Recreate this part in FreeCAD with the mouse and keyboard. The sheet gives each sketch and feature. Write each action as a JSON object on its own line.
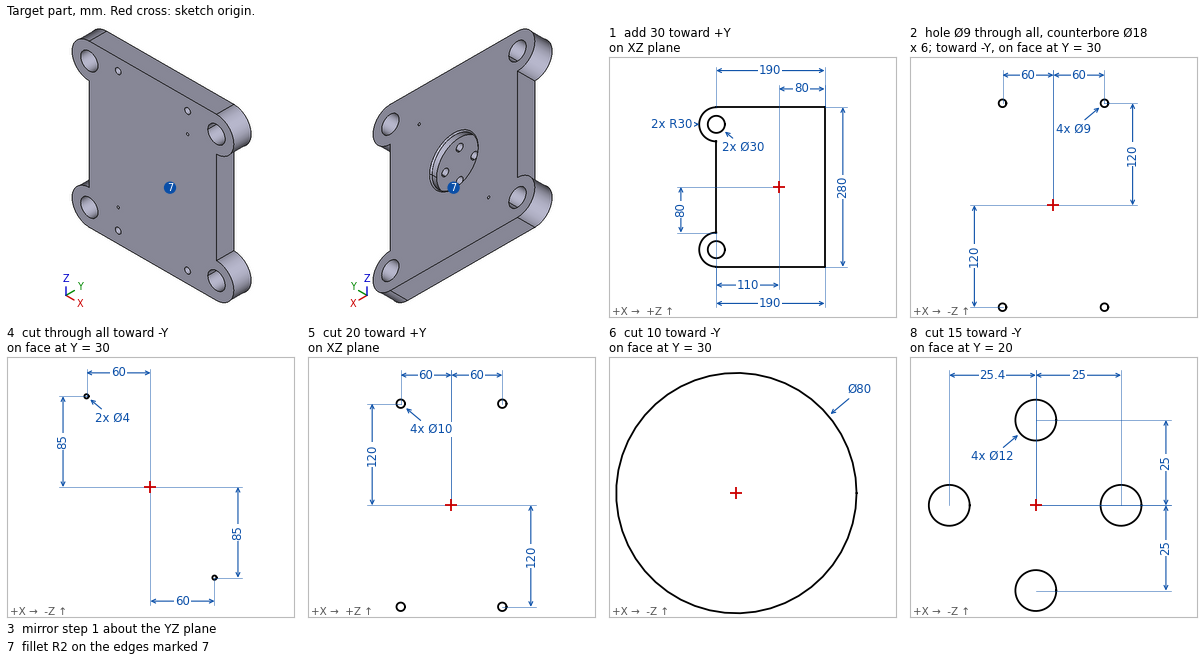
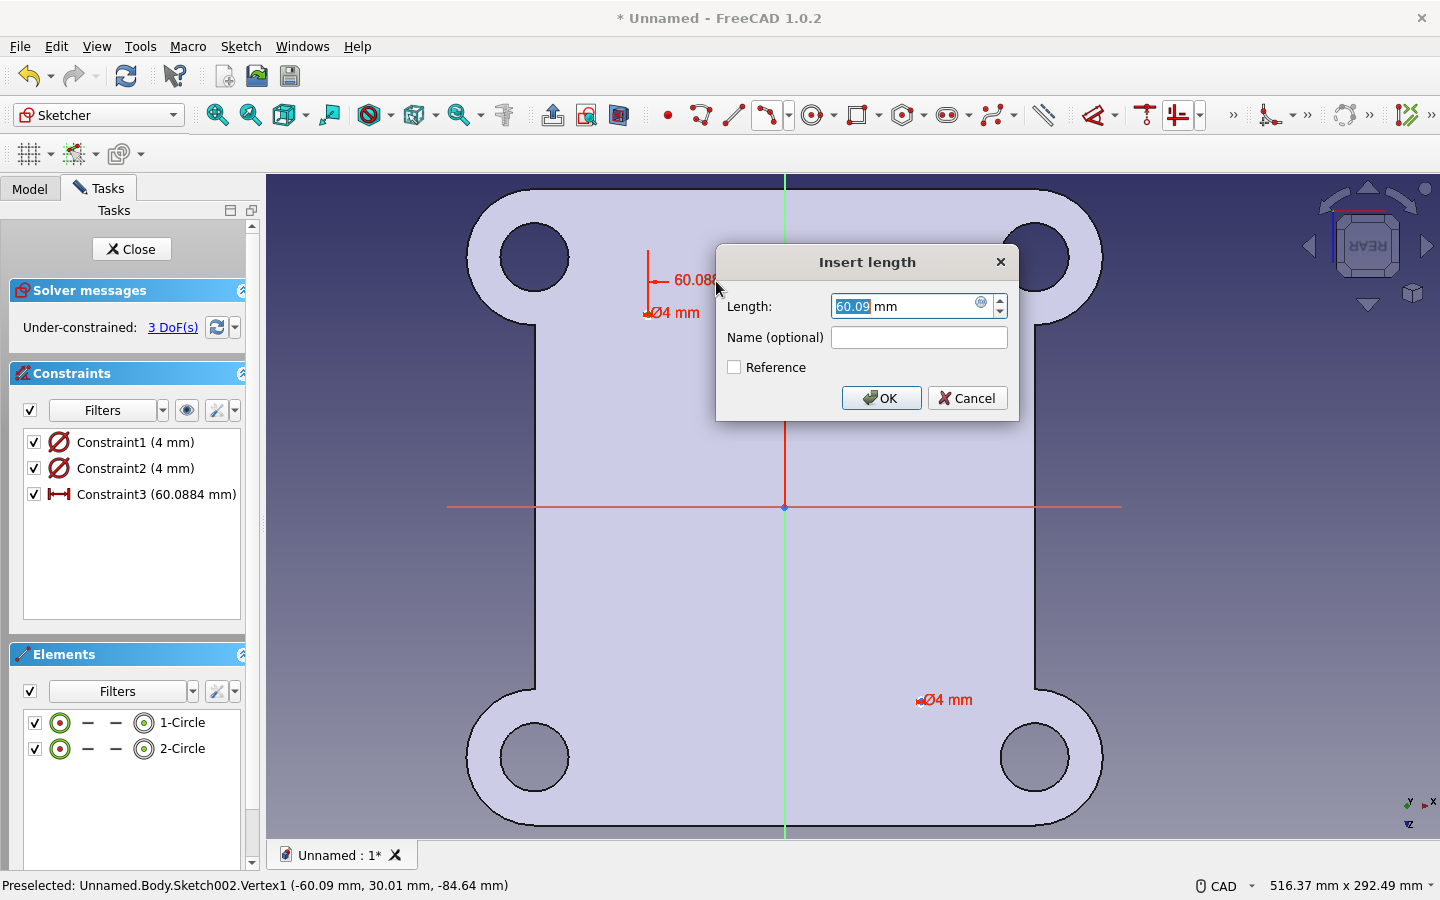
{"action": "type", "text": "60"}
{"action": "key", "text": "Return"}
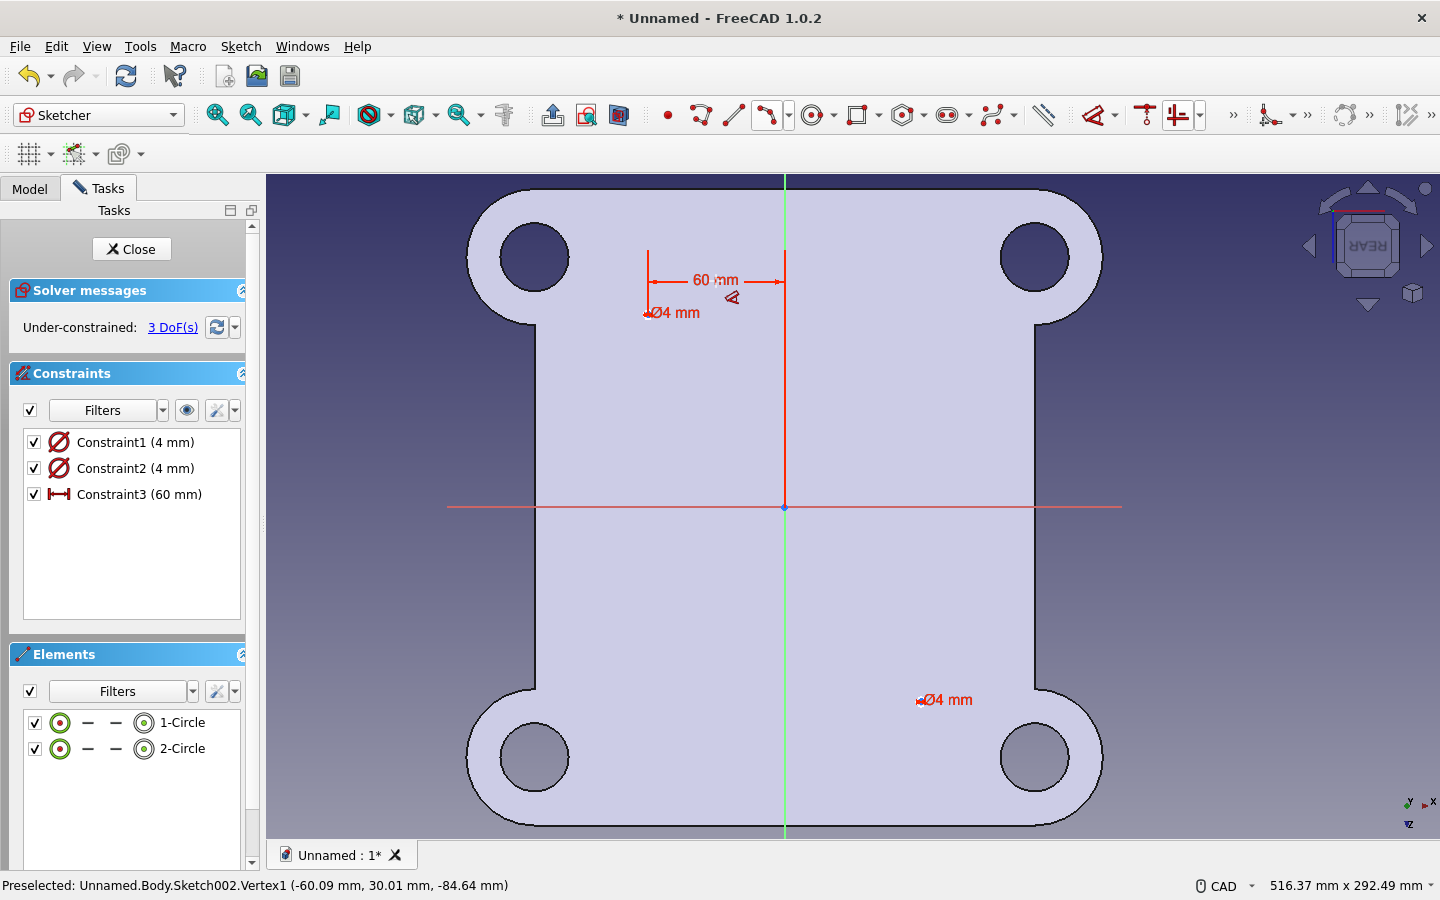
{"action": "left_click", "coordinate": [648, 315]}
{"action": "left_click", "coordinate": [614, 411]}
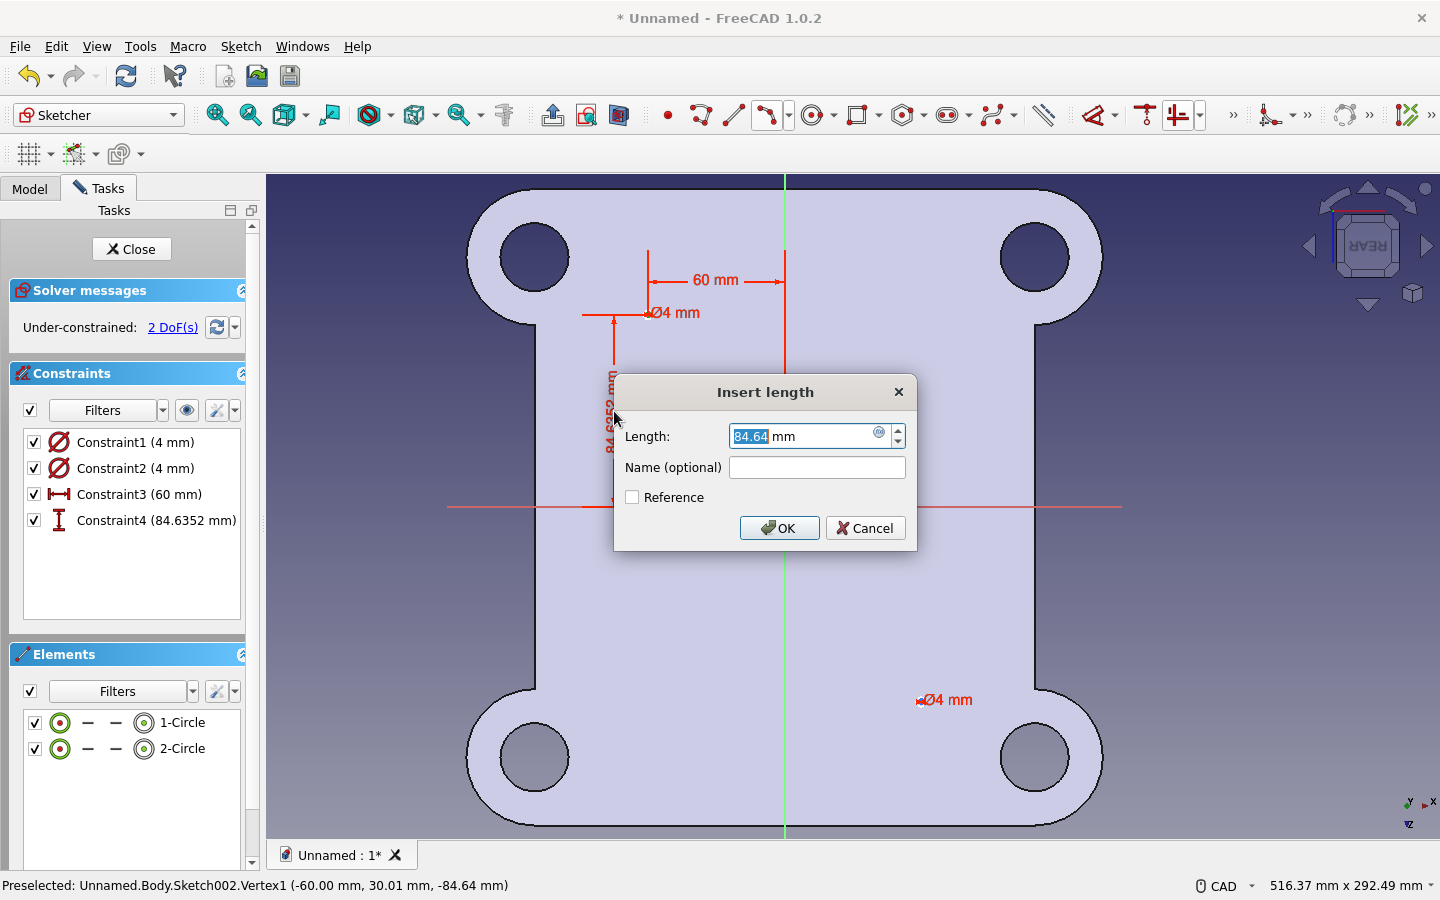
{"action": "type", "text": "85"}
{"action": "key", "text": "Return"}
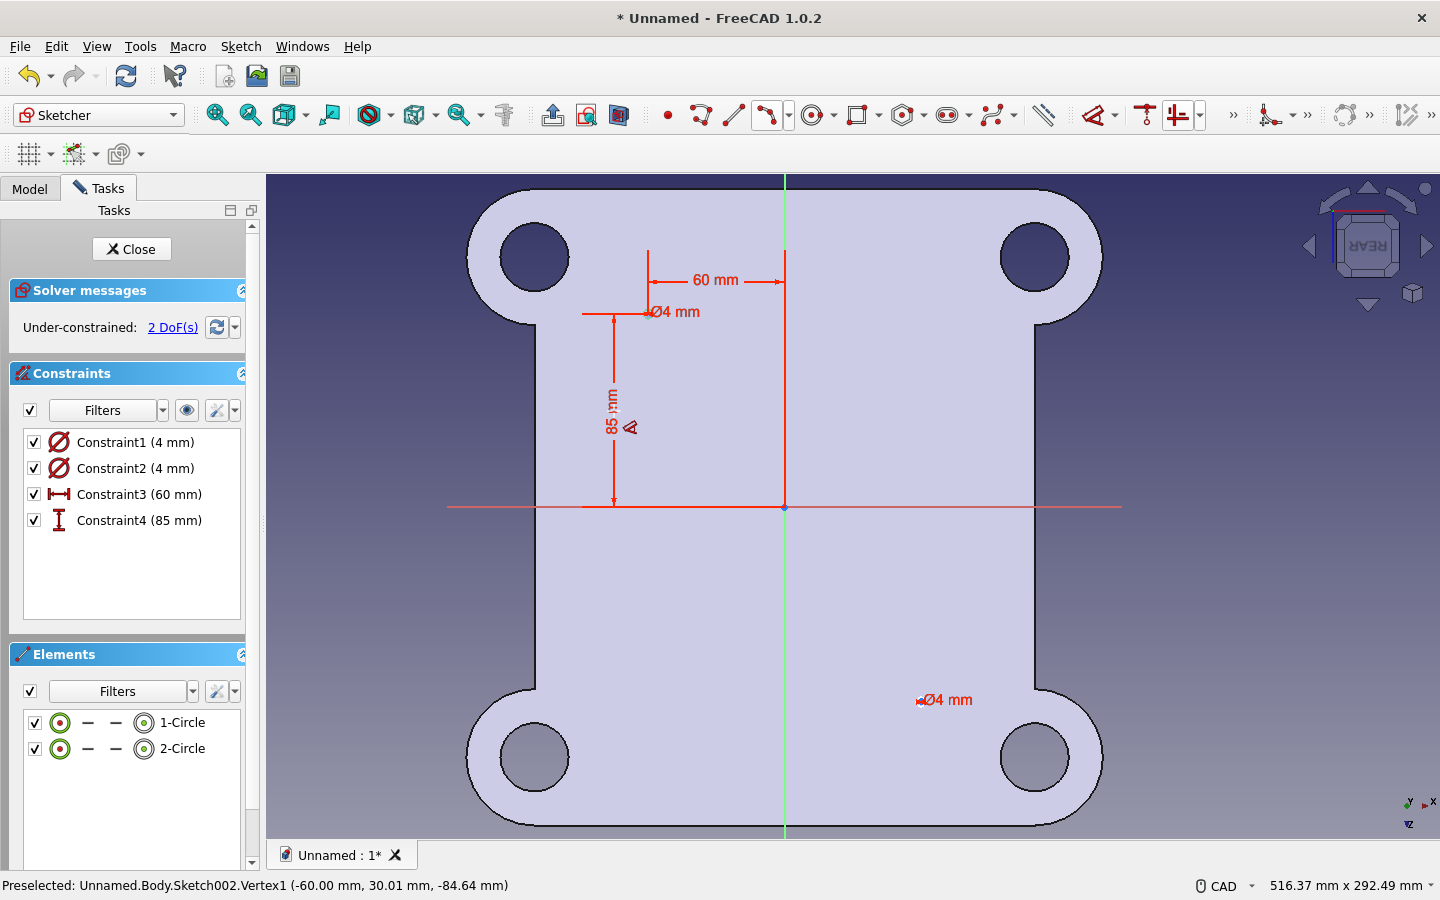
{"action": "left_click", "coordinate": [921, 702]}
{"action": "left_click", "coordinate": [853, 736]}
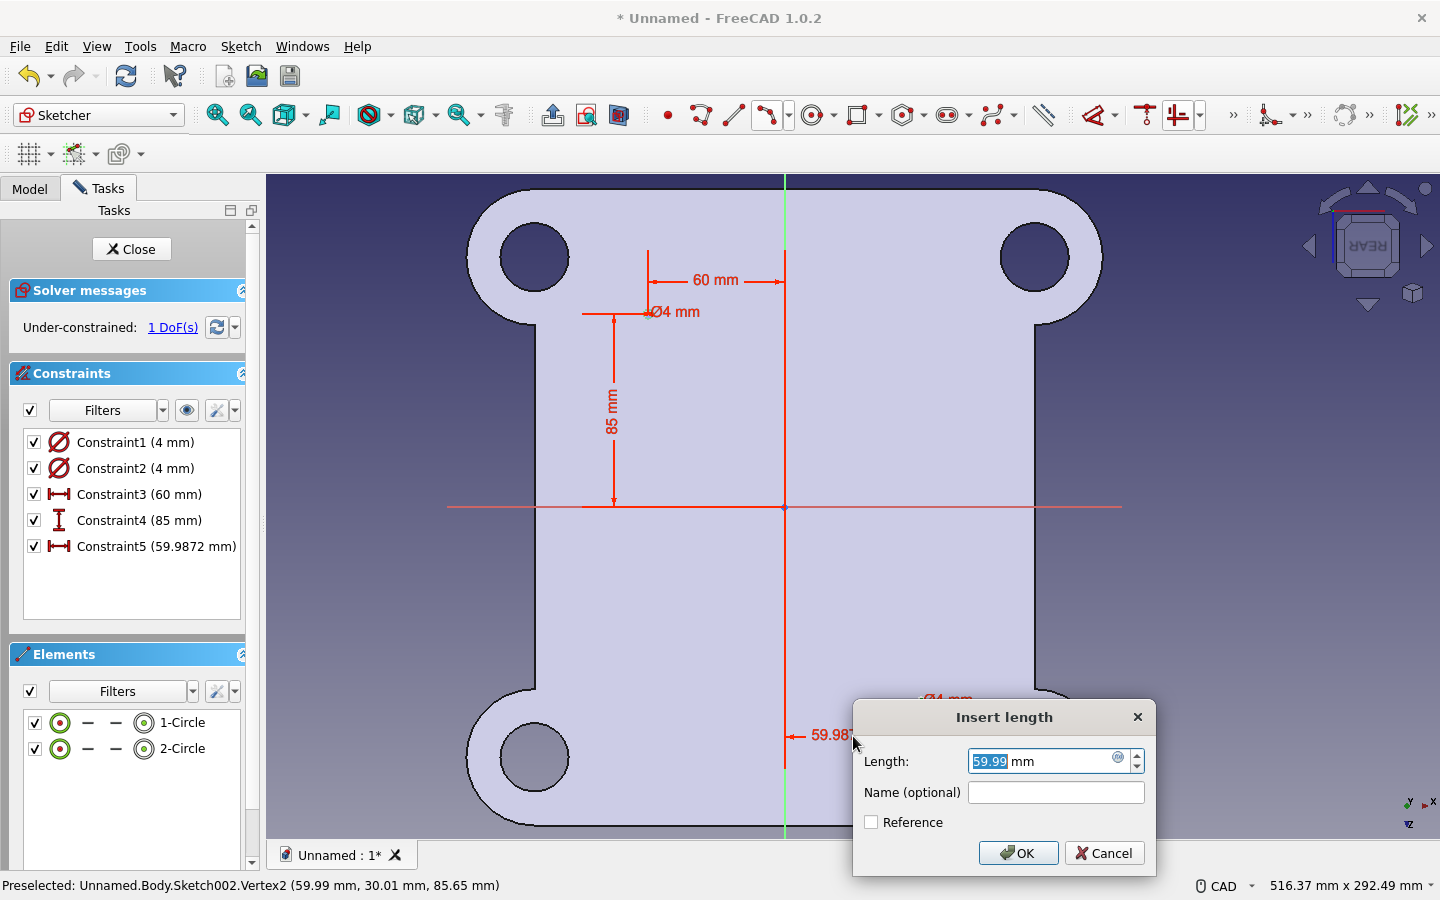
{"action": "type", "text": "60"}
{"action": "key", "text": "Return"}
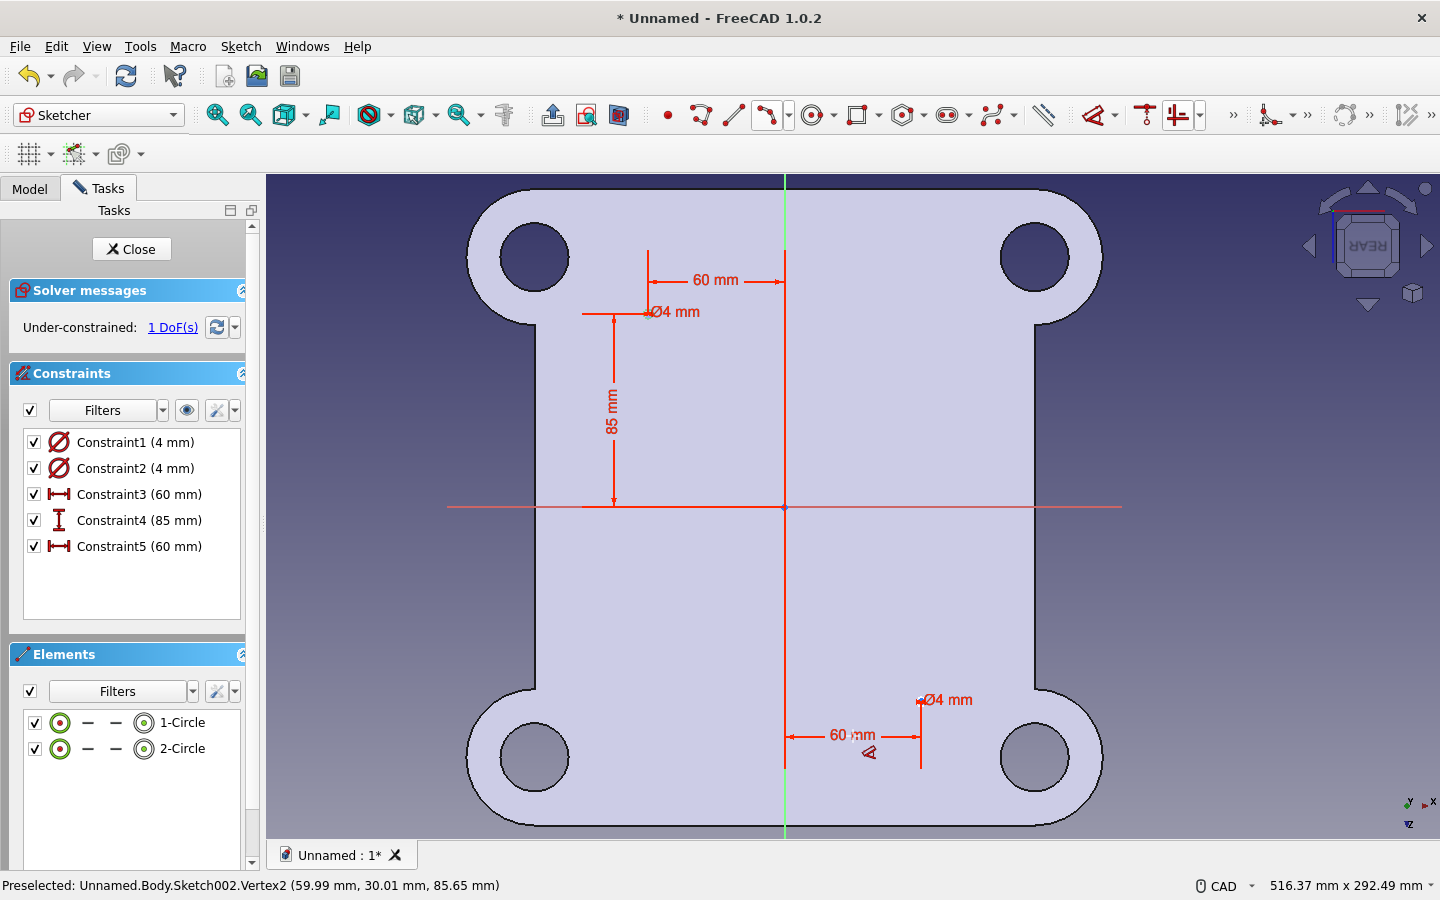
{"action": "left_click", "coordinate": [921, 702]}
{"action": "left_click", "coordinate": [955, 605]}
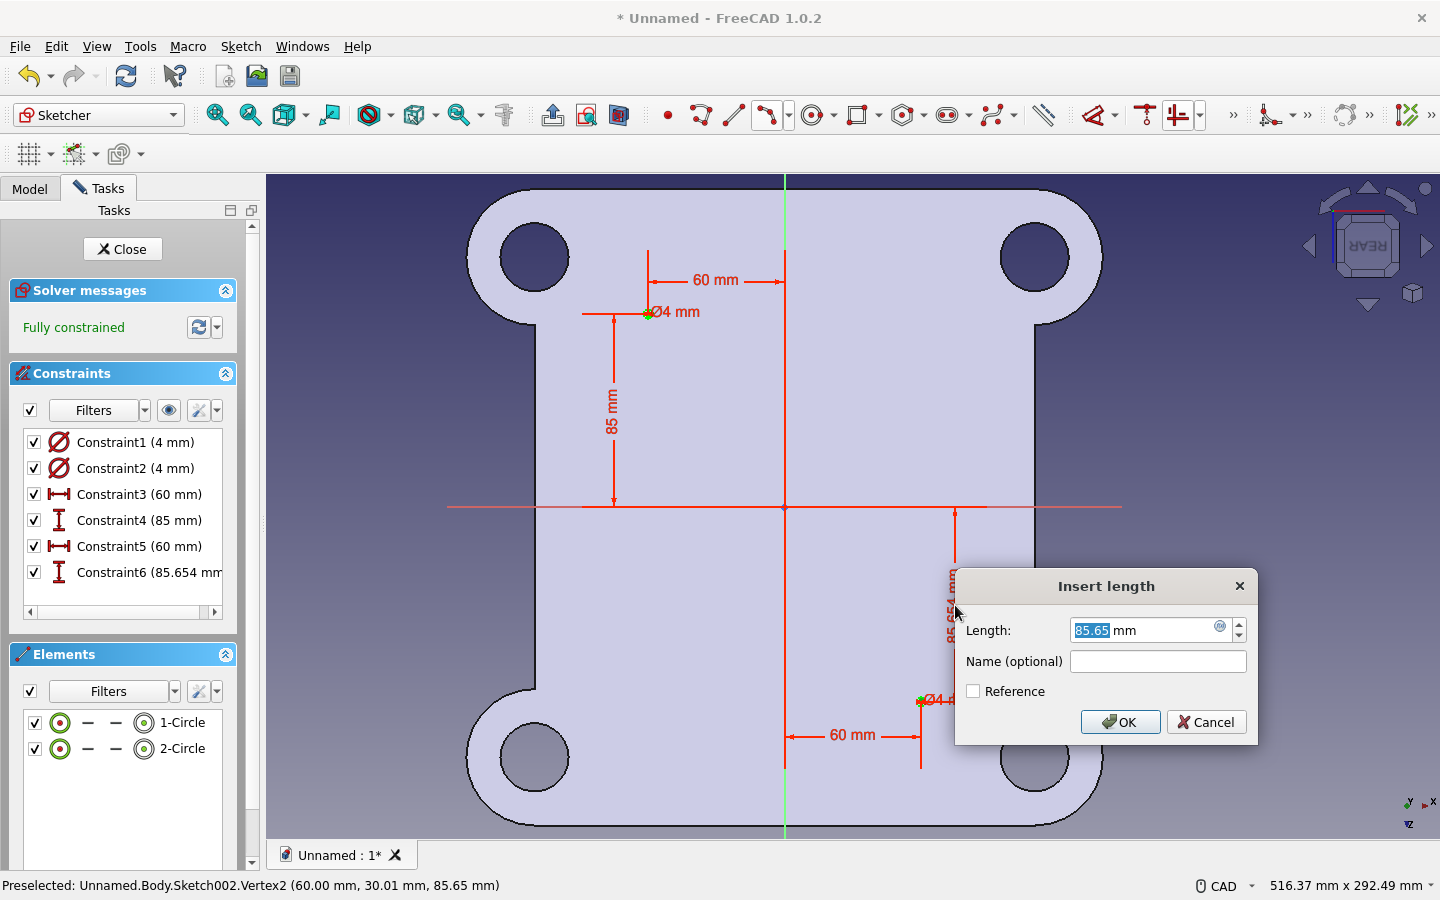
{"action": "type", "text": "85"}
{"action": "key", "text": "Return"}
{"action": "key", "text": "Escape"}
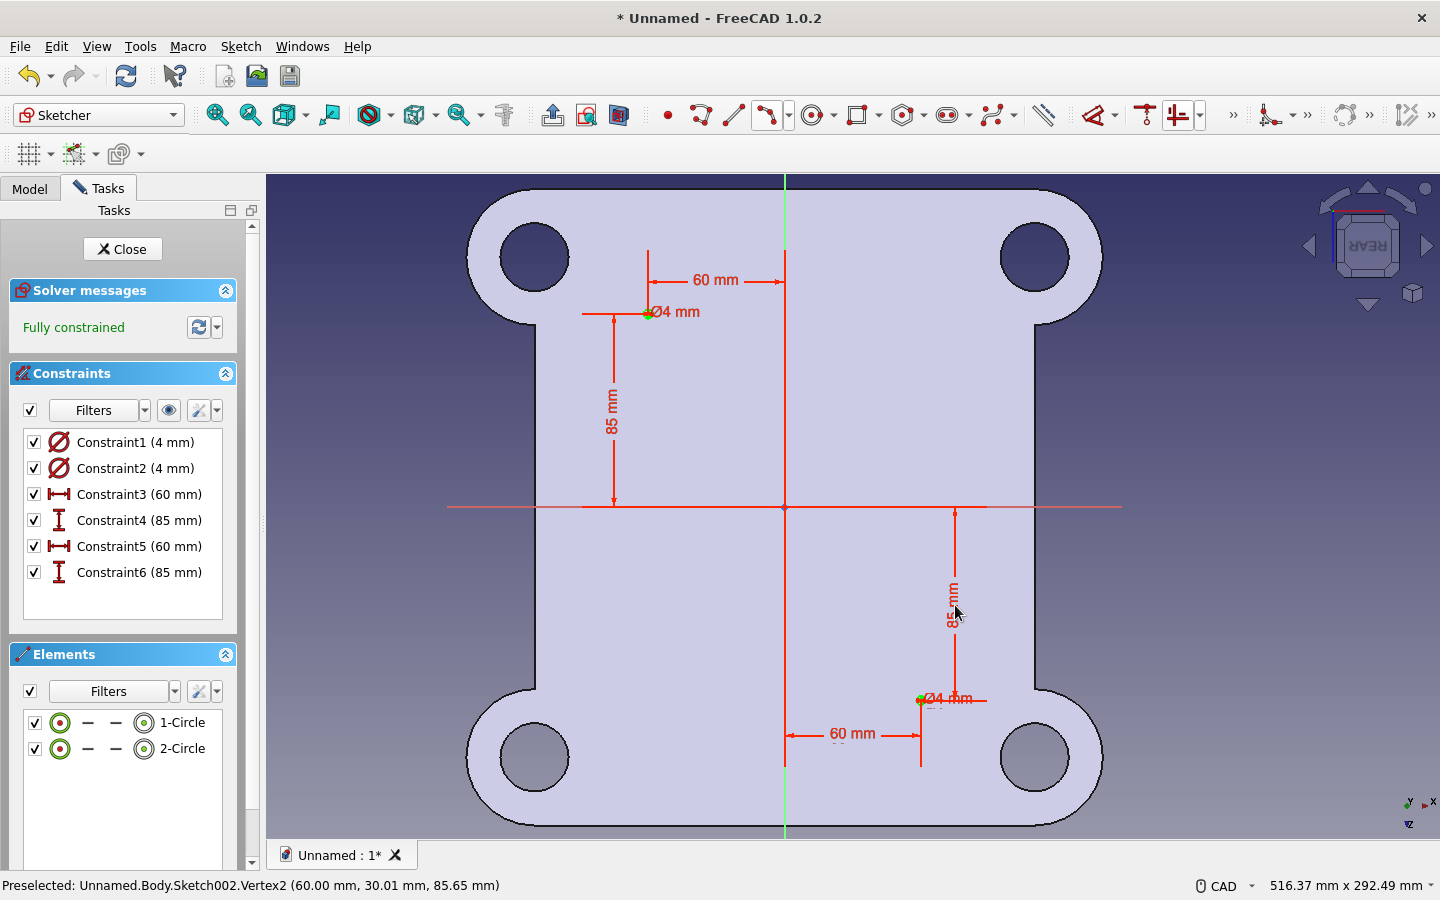
{"action": "left_click", "coordinate": [123, 249]}